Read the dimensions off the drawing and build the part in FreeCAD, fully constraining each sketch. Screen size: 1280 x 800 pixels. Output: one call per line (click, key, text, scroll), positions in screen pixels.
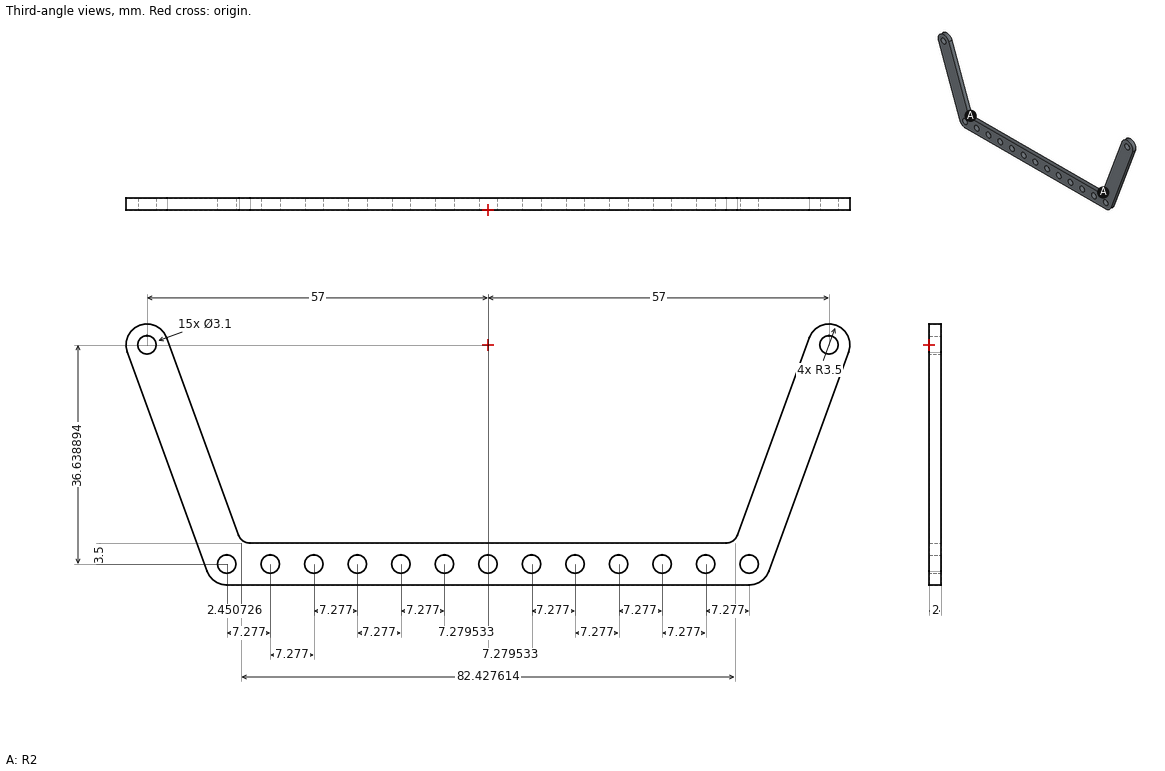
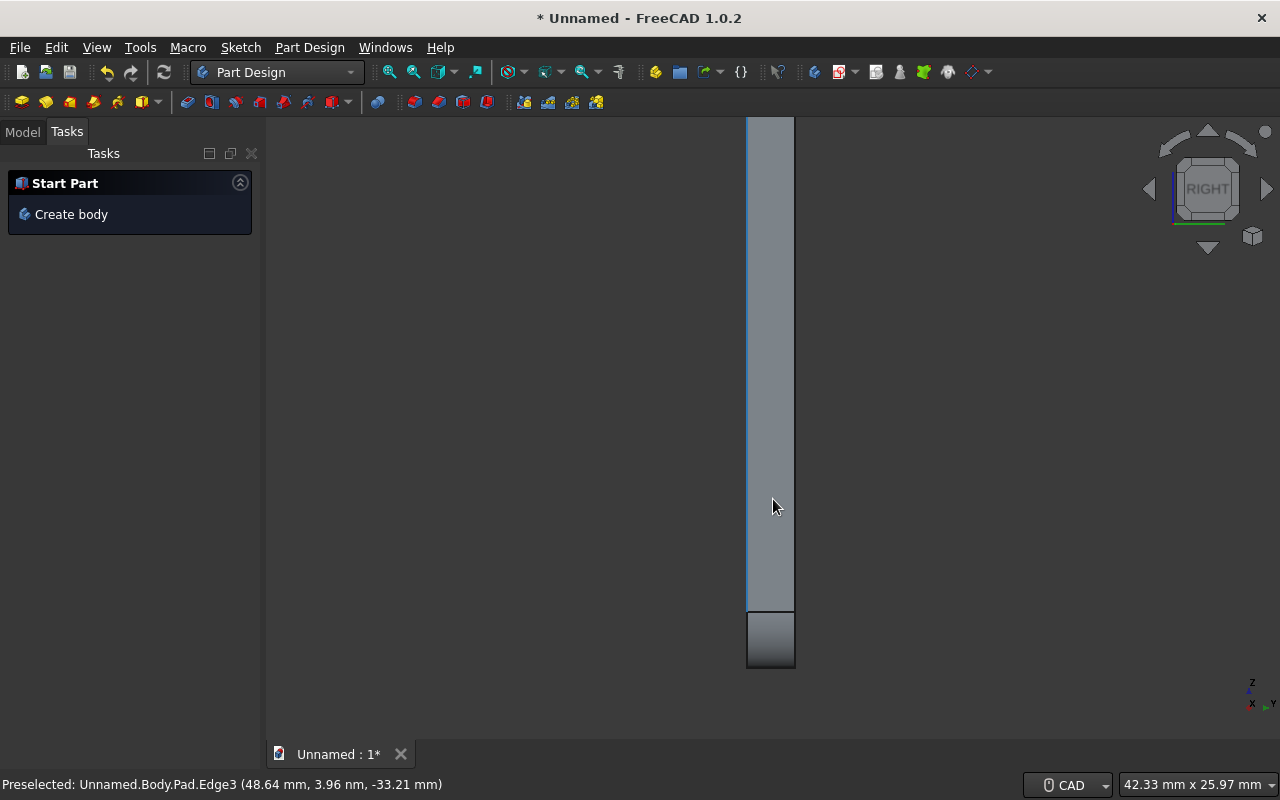
click(390, 72)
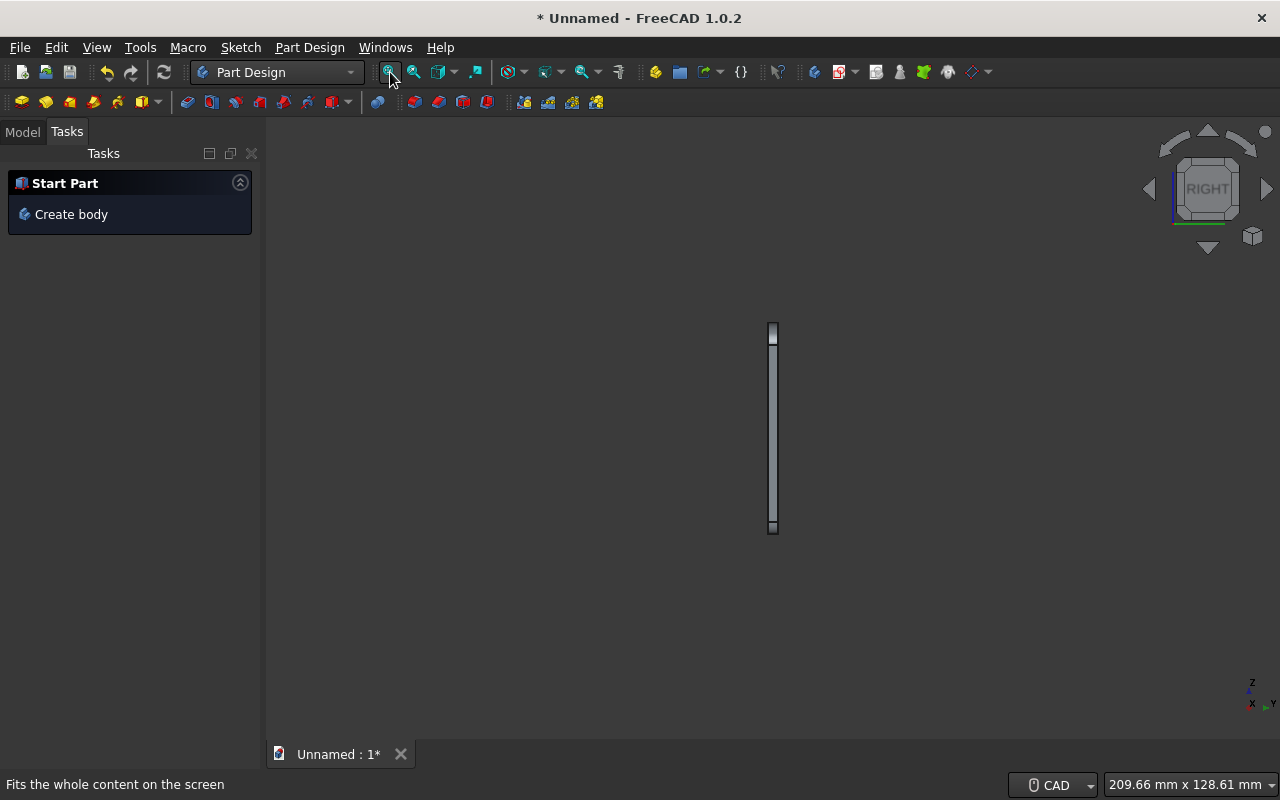
key(5)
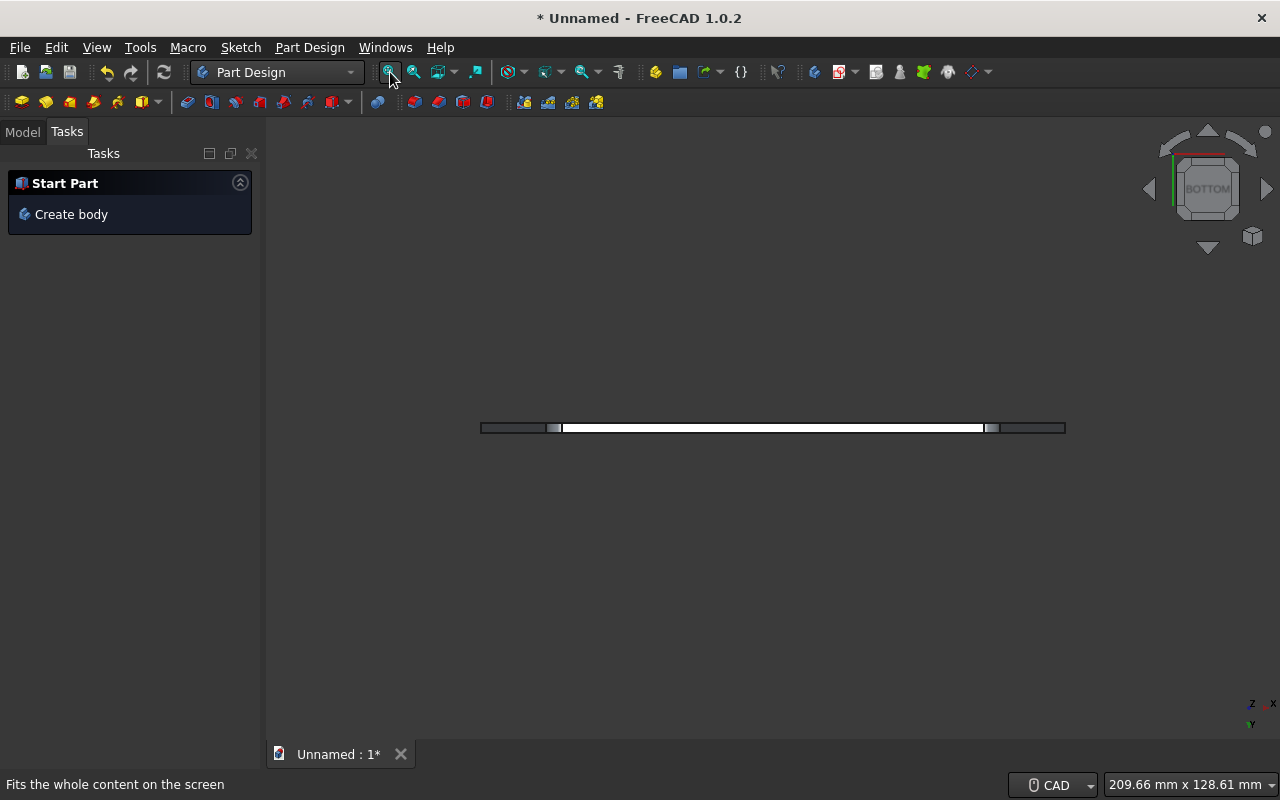
scroll(574, 427, up, 8)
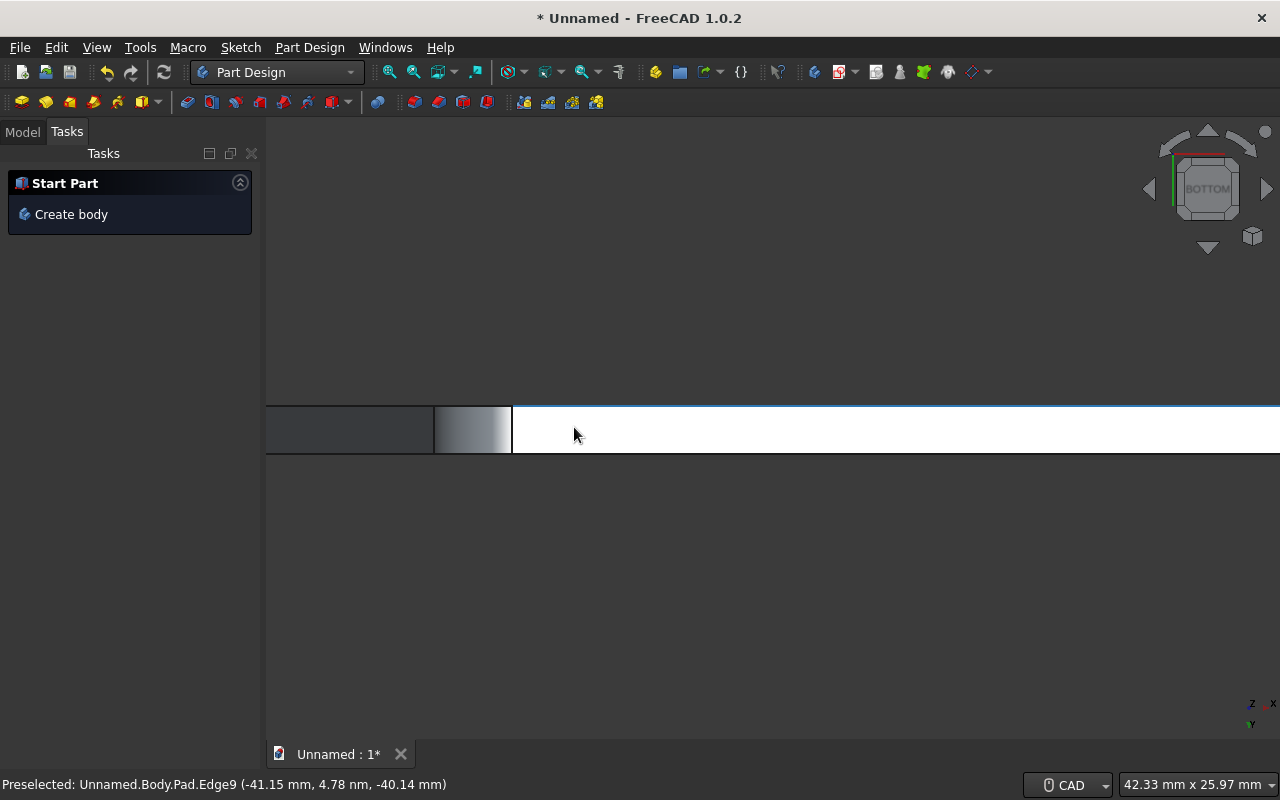
click(390, 72)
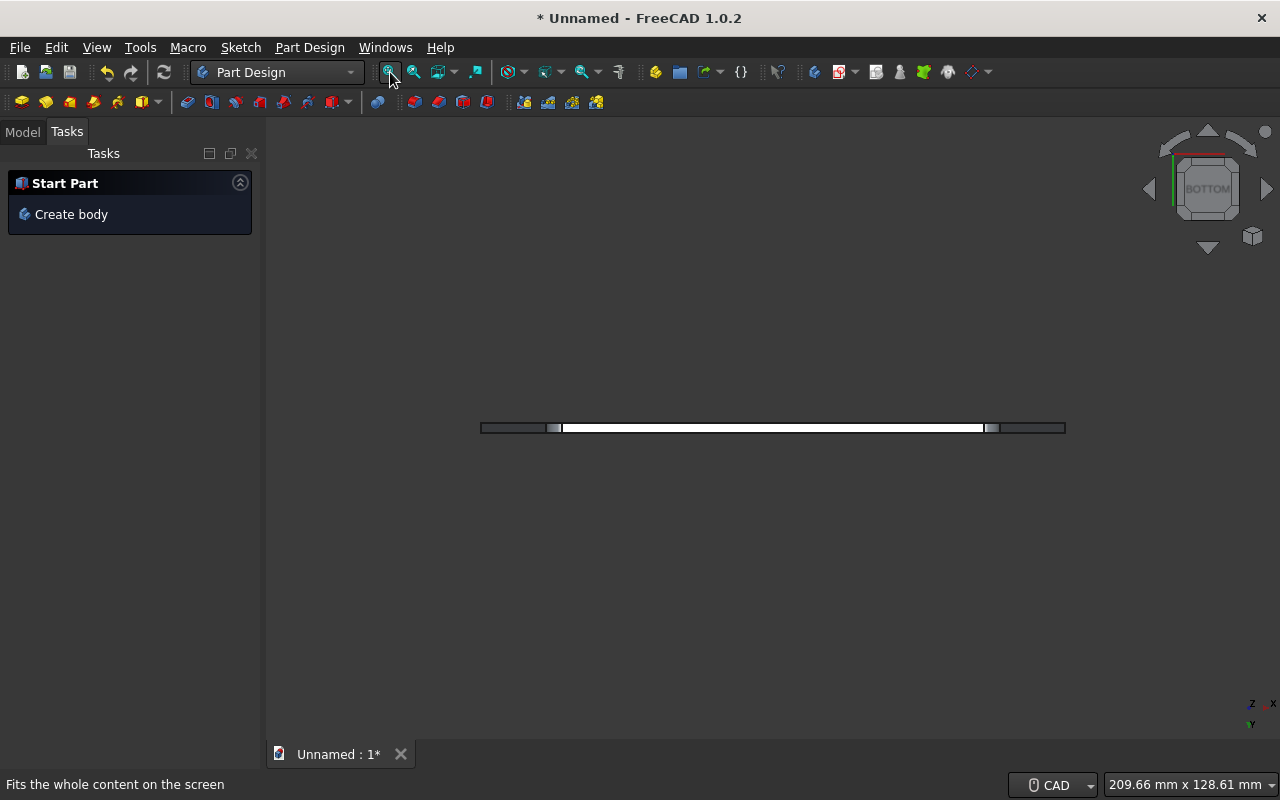
key(4)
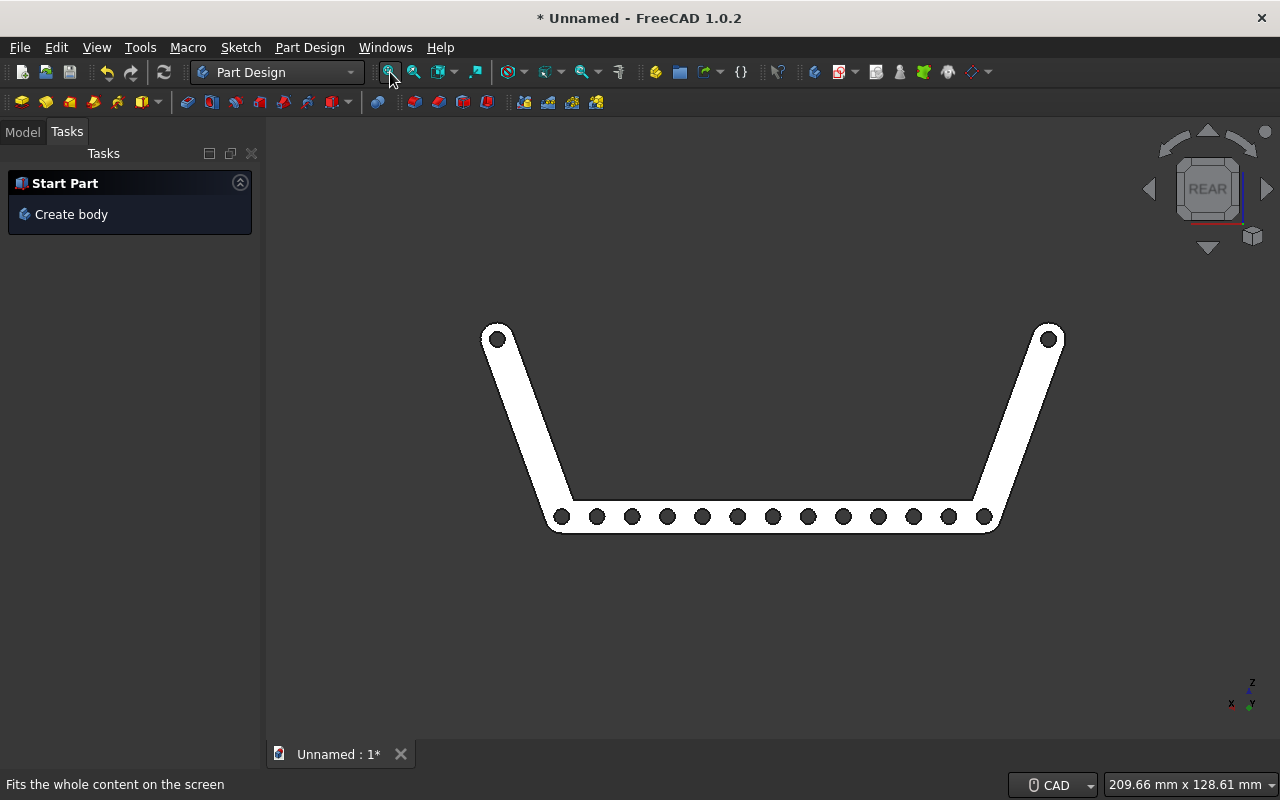
scroll(972, 499, up, 8)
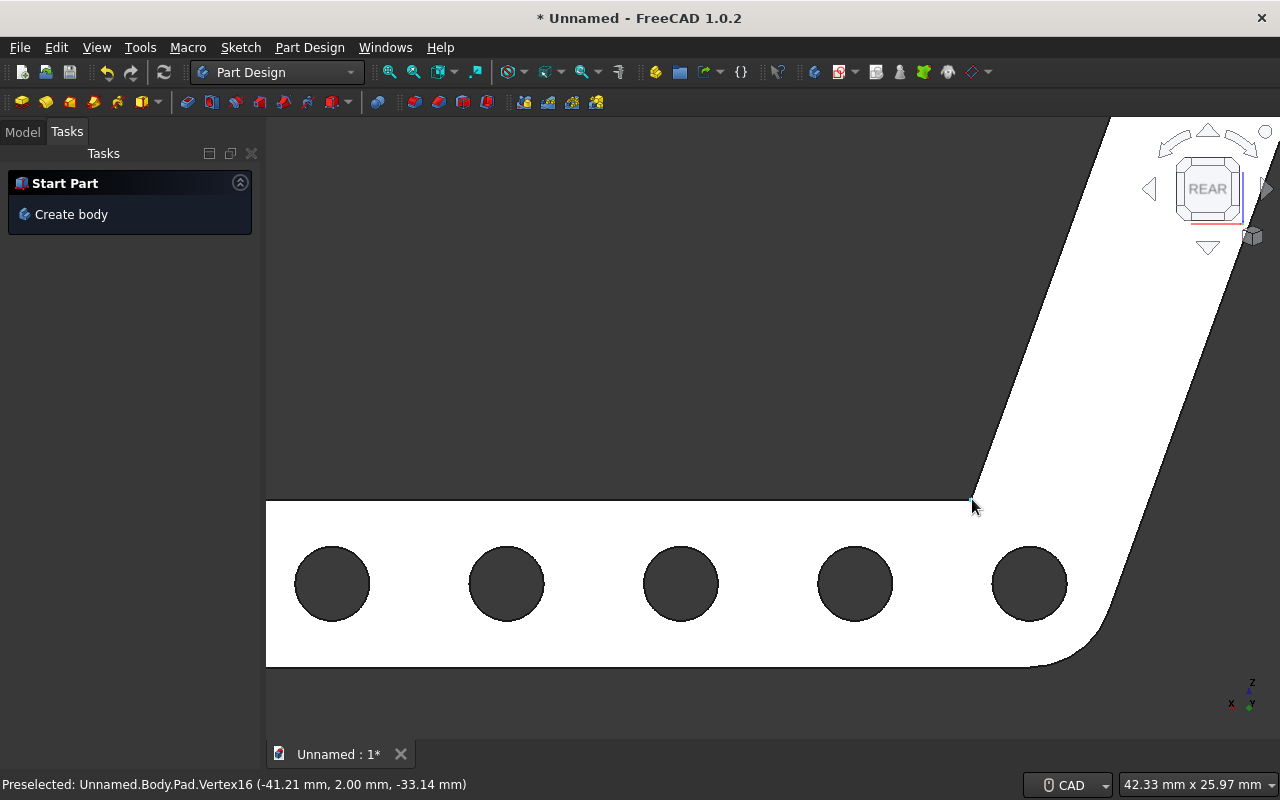
click(390, 72)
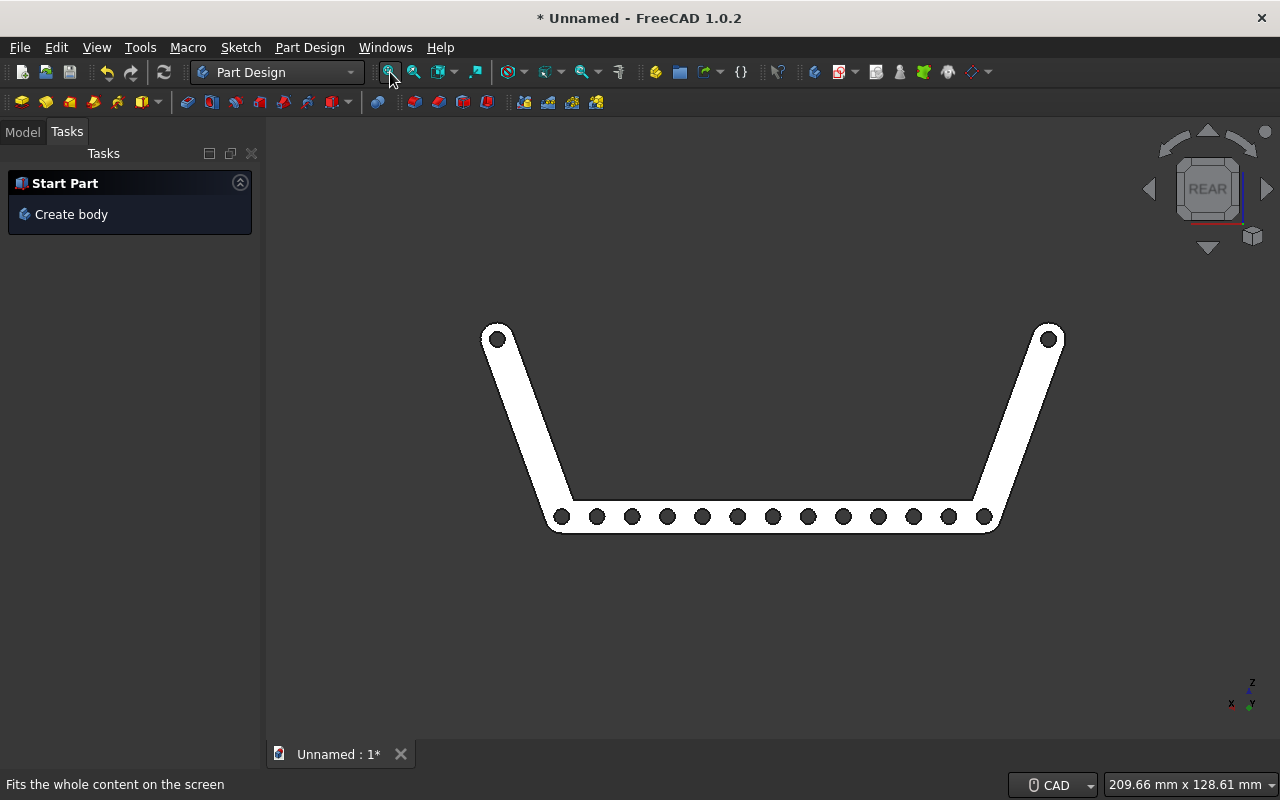
key(6)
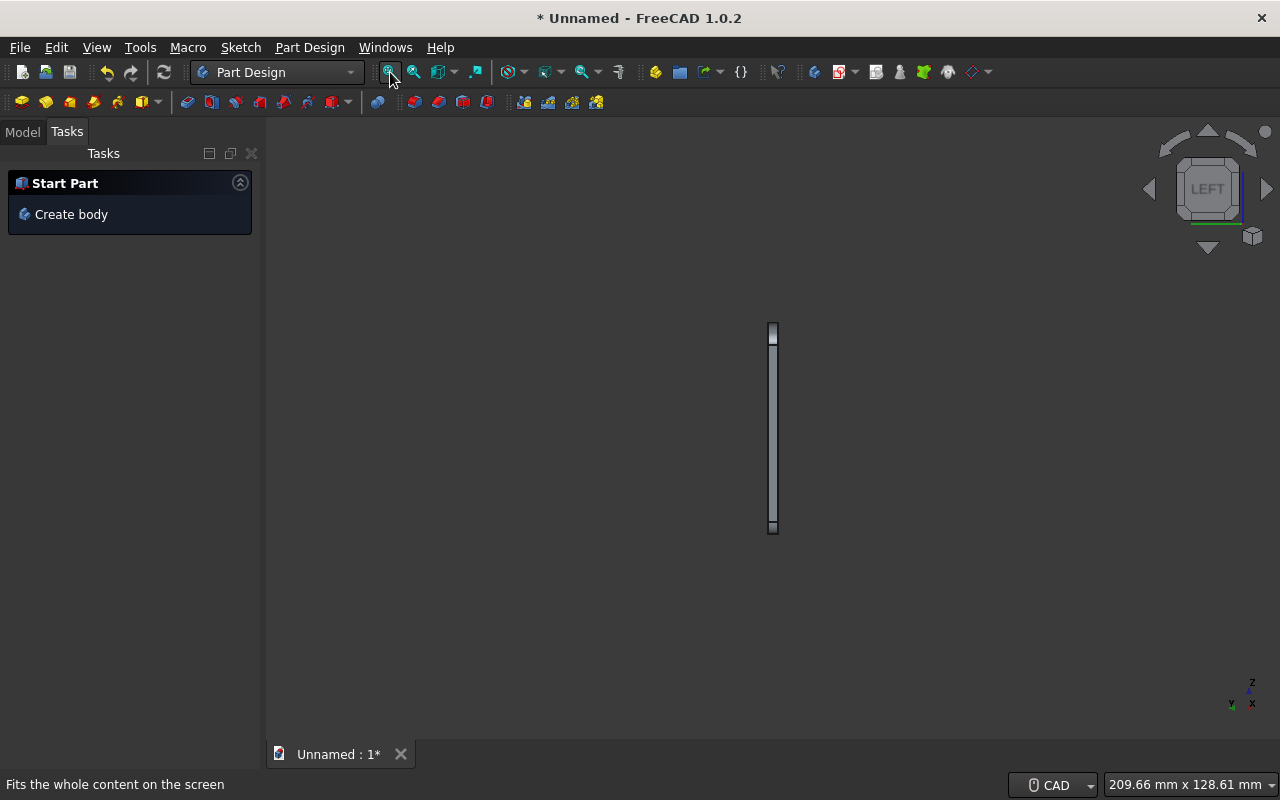
key(v)
key(f)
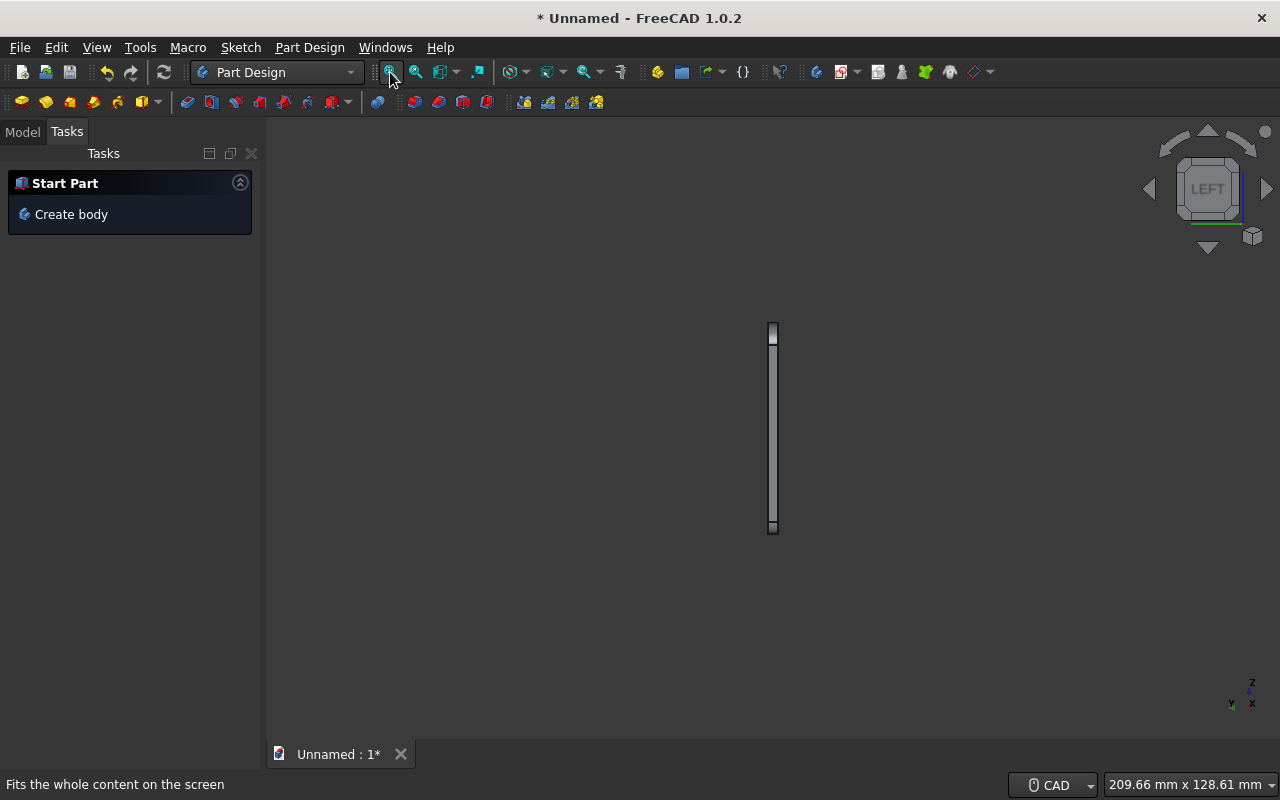
scroll(773, 499, up, 8)